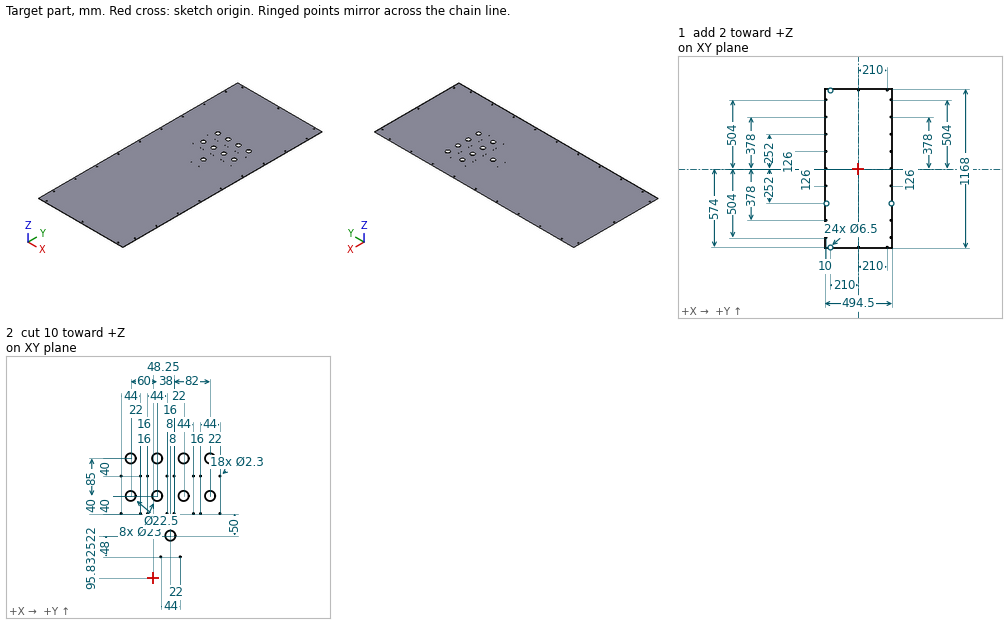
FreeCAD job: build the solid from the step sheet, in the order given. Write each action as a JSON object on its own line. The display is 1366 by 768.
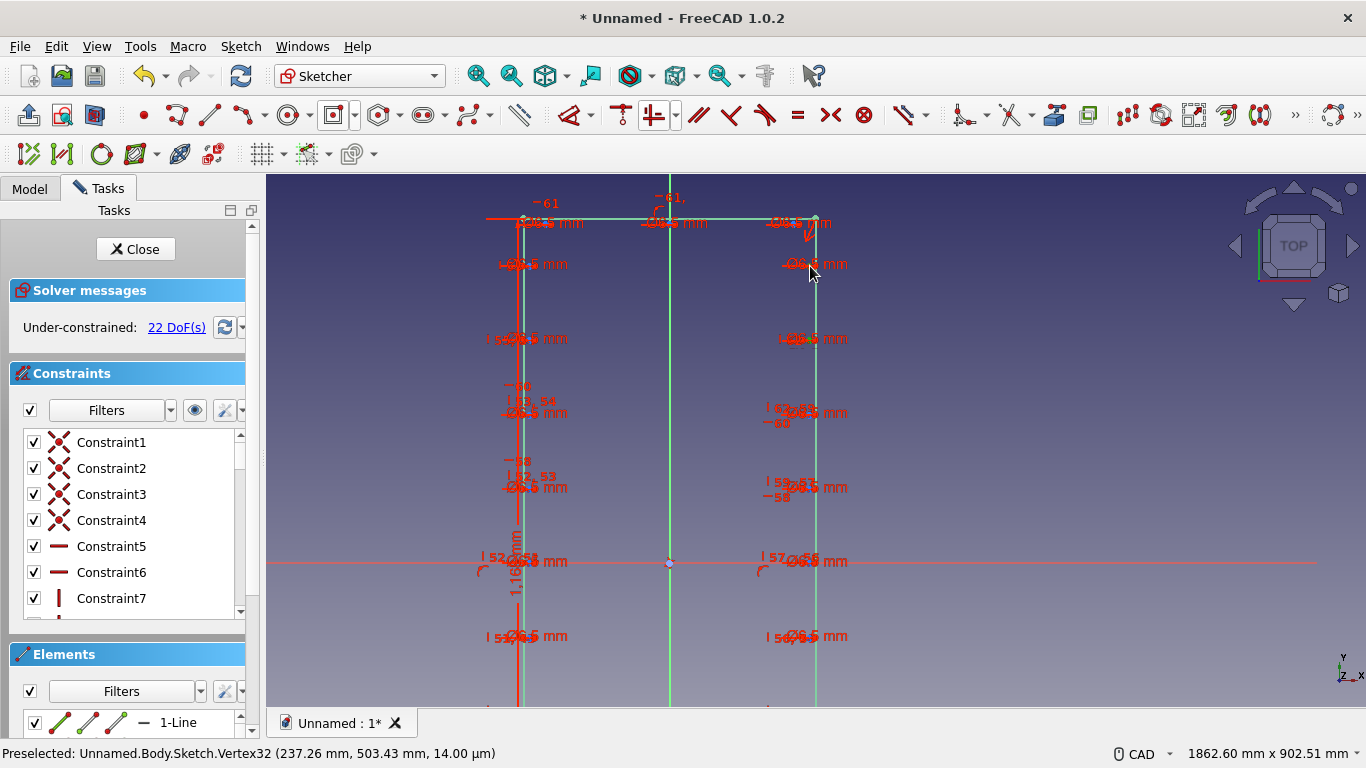
{"action": "key", "text": "v"}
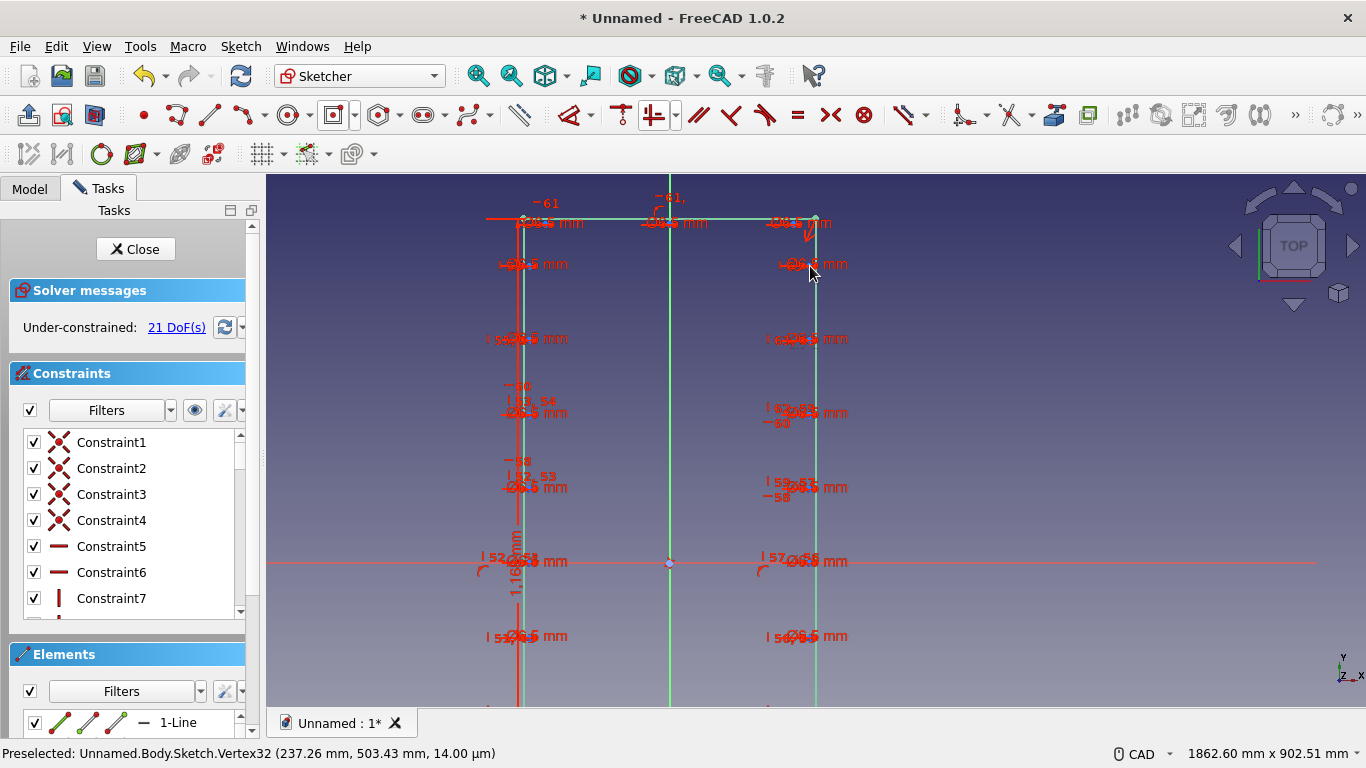
{"action": "left_click", "coordinate": [670, 225]}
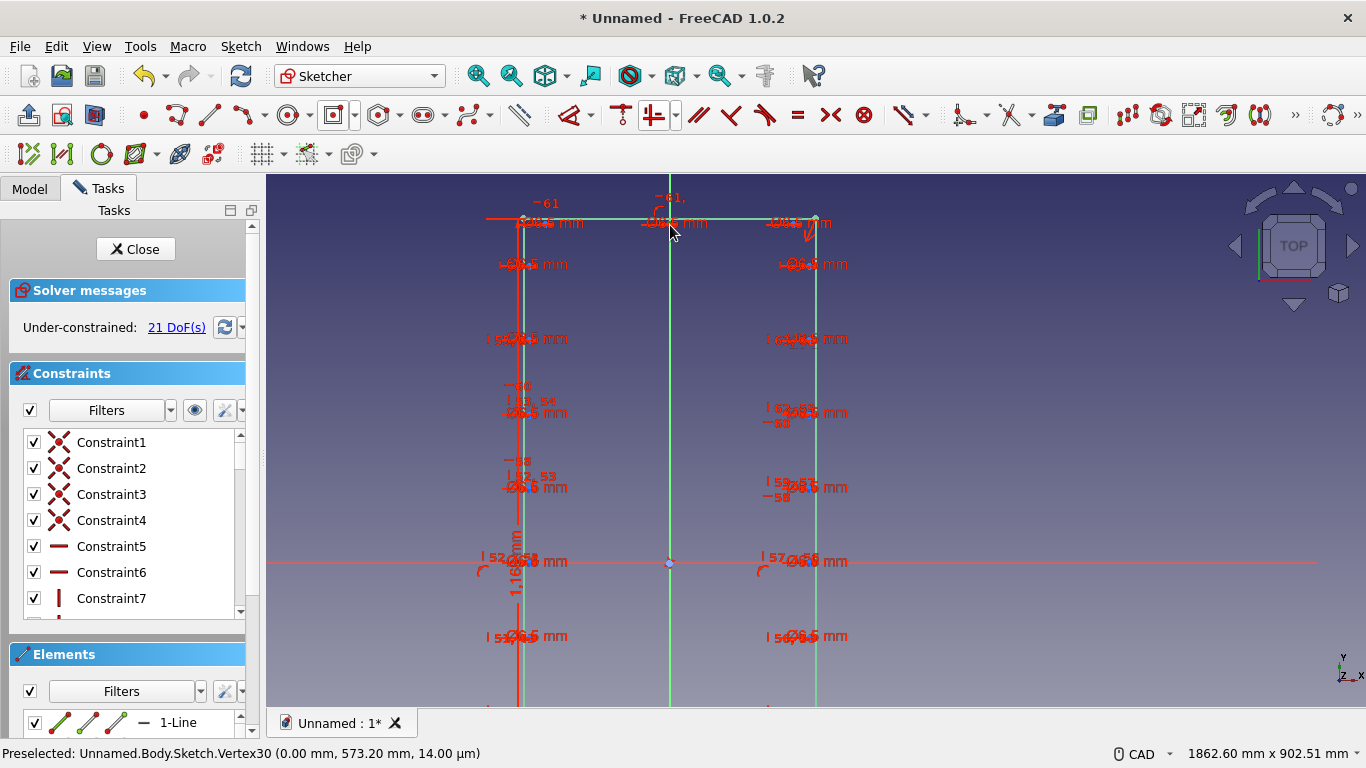
{"action": "left_click", "coordinate": [794, 225]}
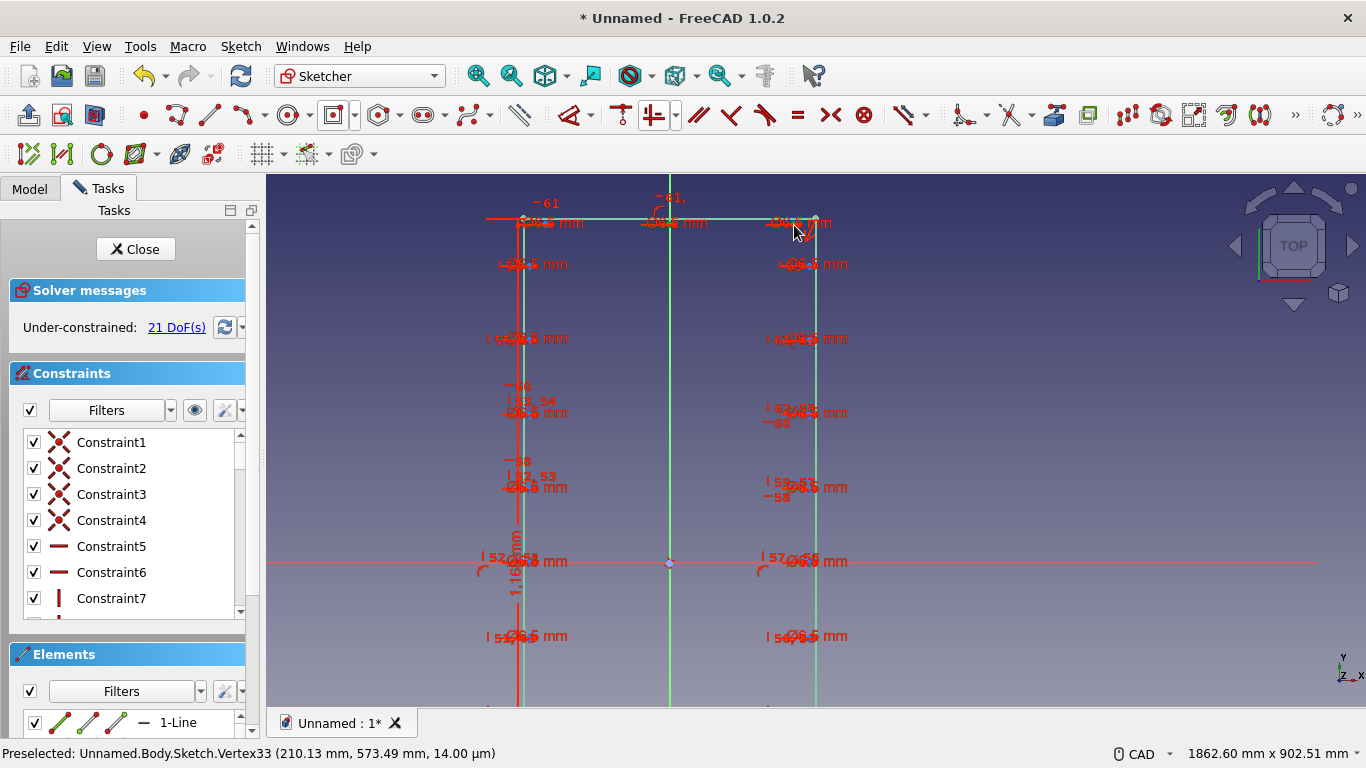
{"action": "left_click", "coordinate": [676, 116]}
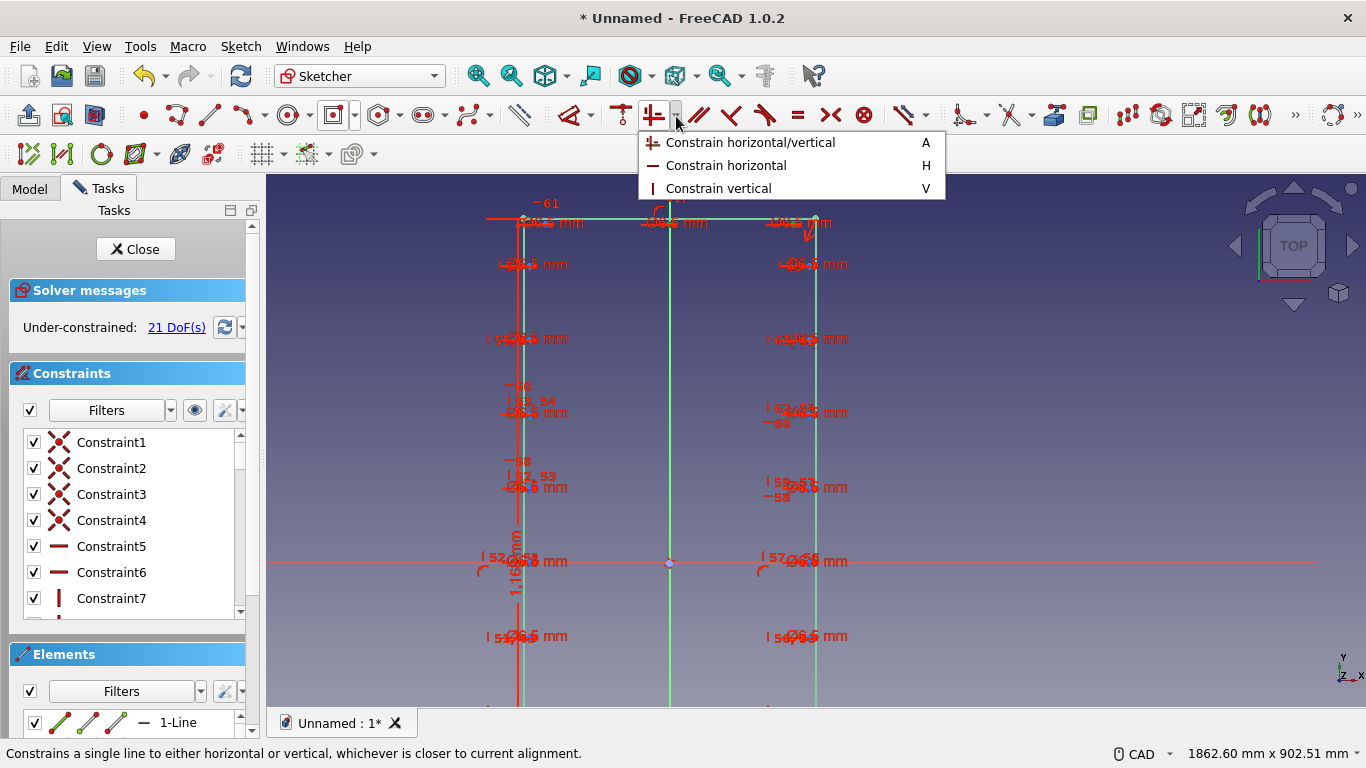
{"action": "left_click", "coordinate": [792, 166]}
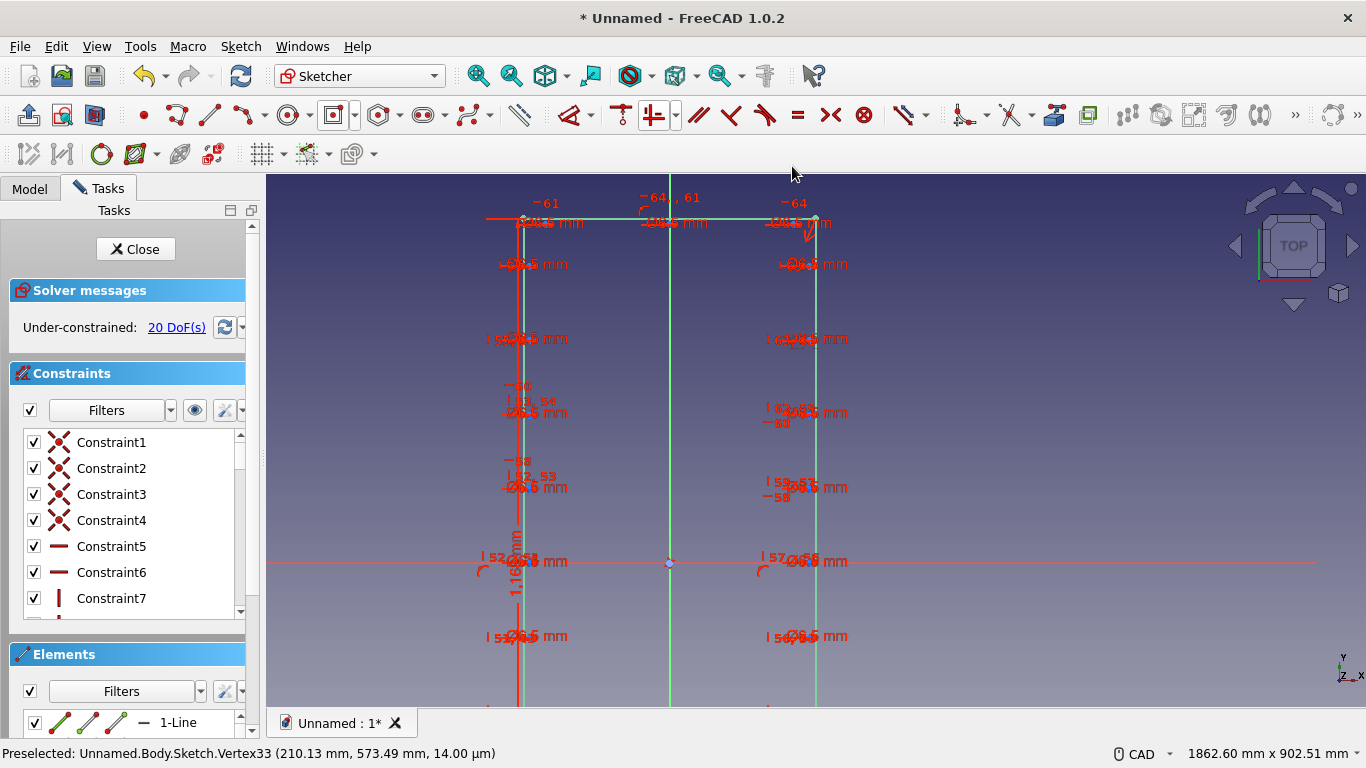
{"action": "scroll", "coordinate": [811, 340], "scroll_direction": "down", "scroll_amount": 4}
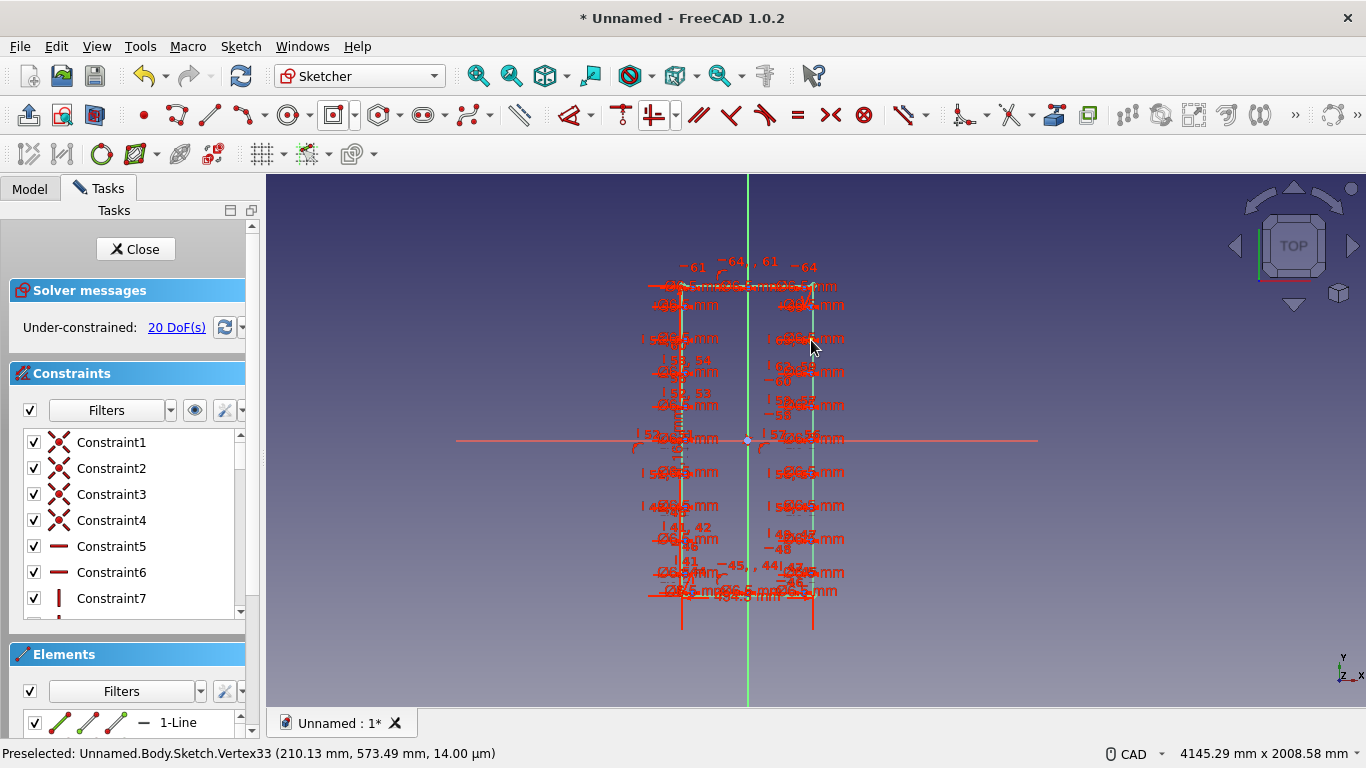
{"action": "left_click", "coordinate": [685, 508]}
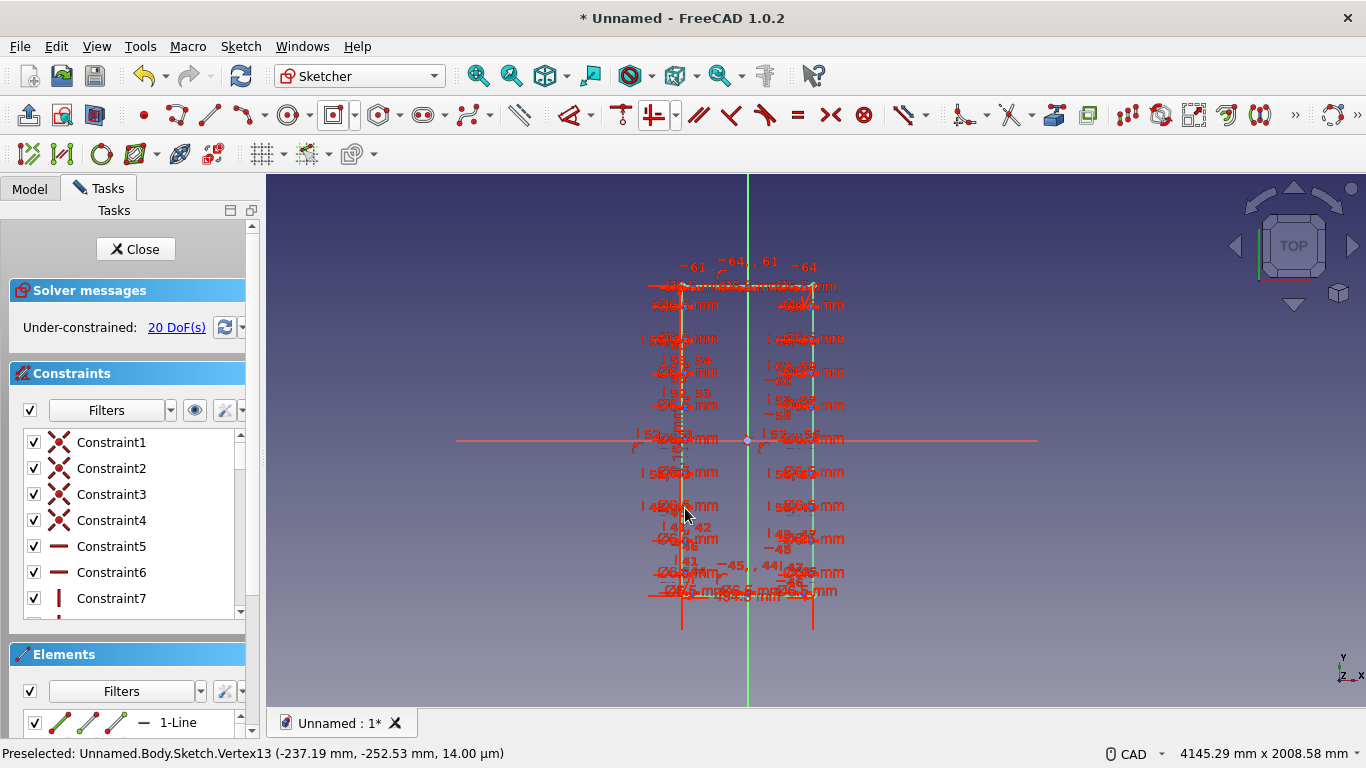
{"action": "left_click", "coordinate": [811, 508]}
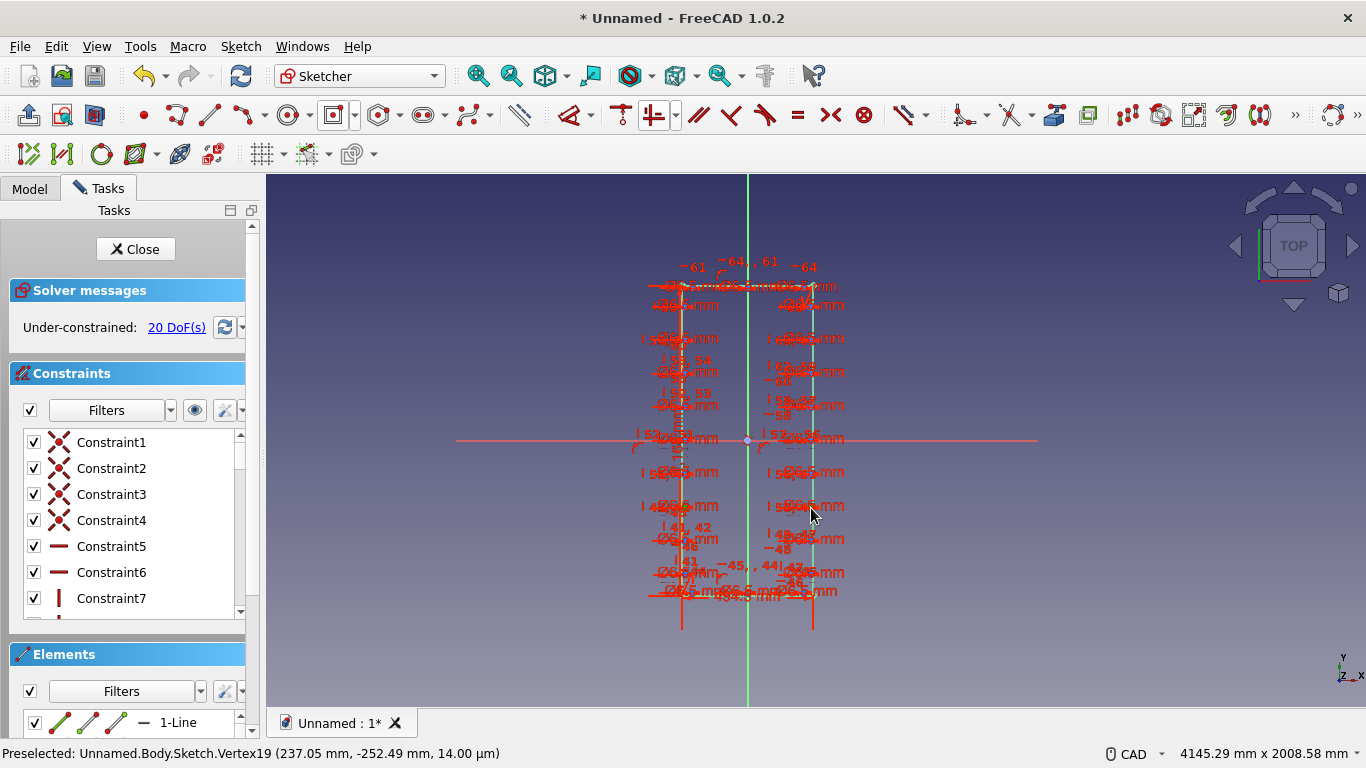
{"action": "left_click", "coordinate": [748, 645]}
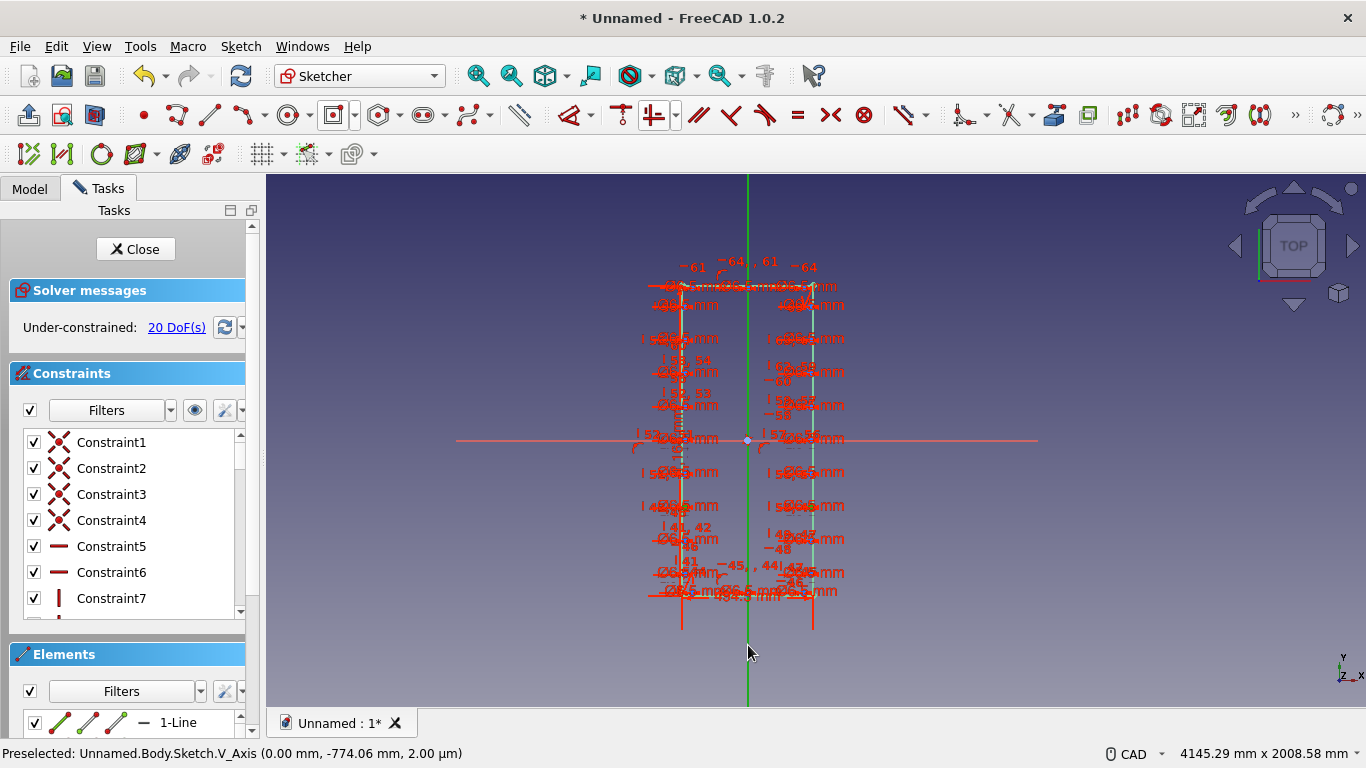
{"action": "left_click", "coordinate": [831, 116]}